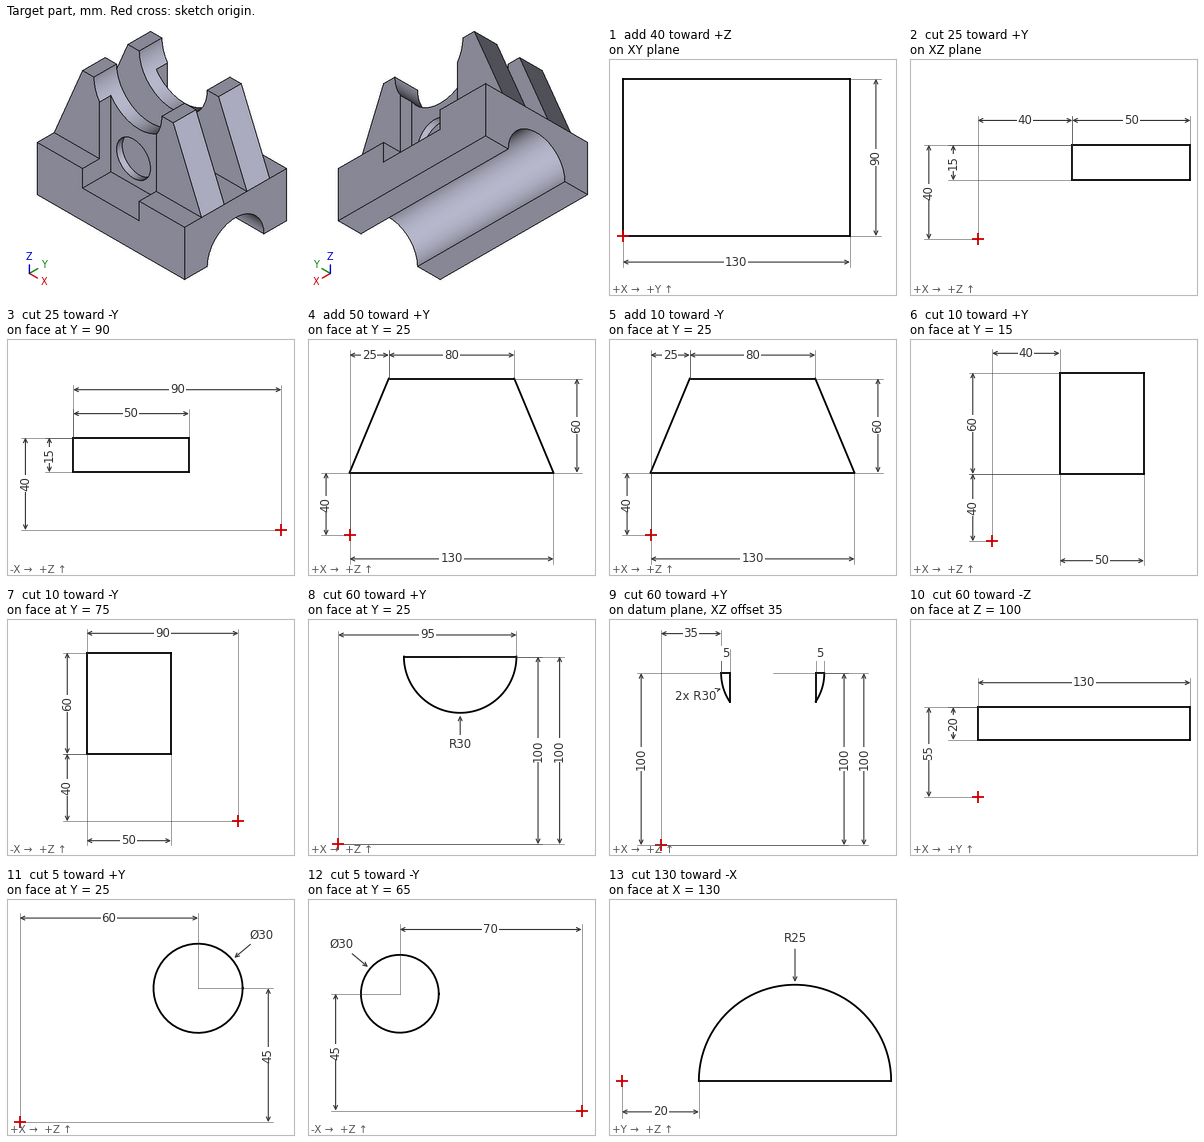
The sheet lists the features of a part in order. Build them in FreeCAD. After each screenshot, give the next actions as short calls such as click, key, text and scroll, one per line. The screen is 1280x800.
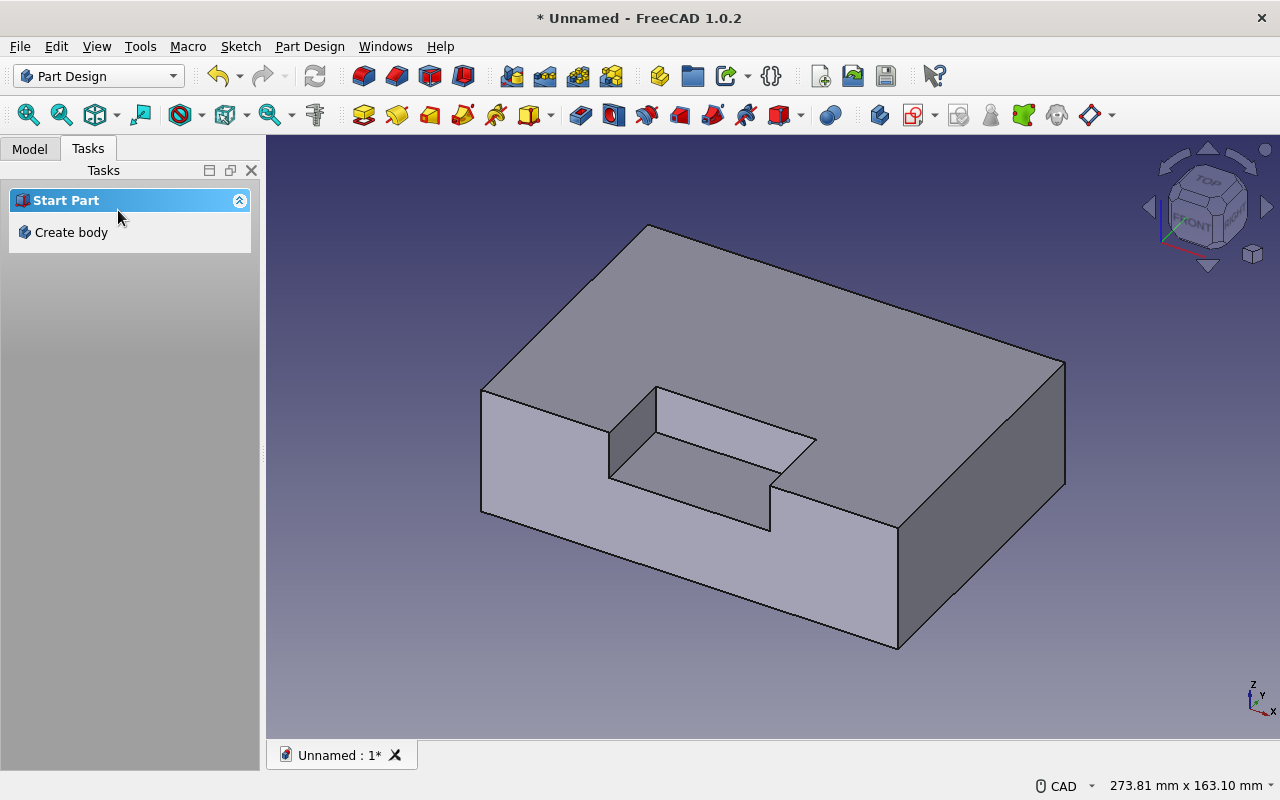
key(4)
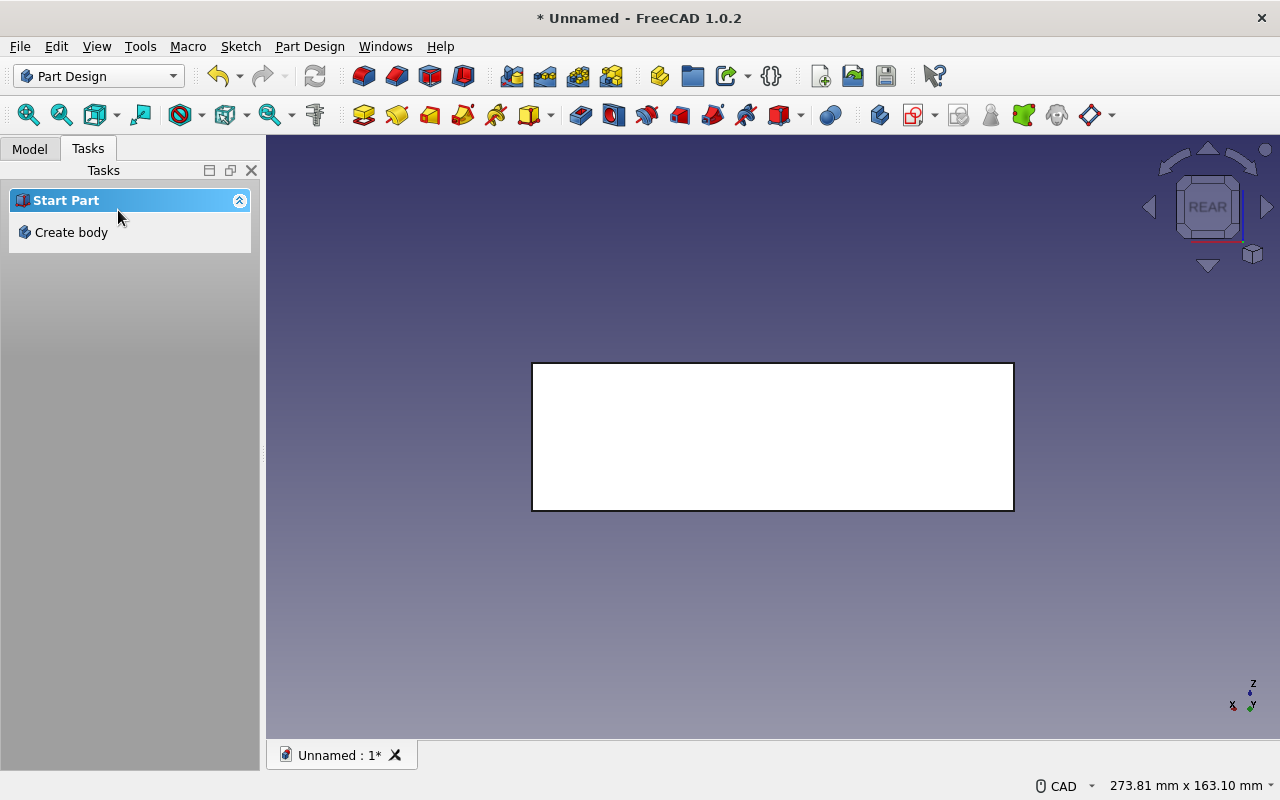
click(635, 436)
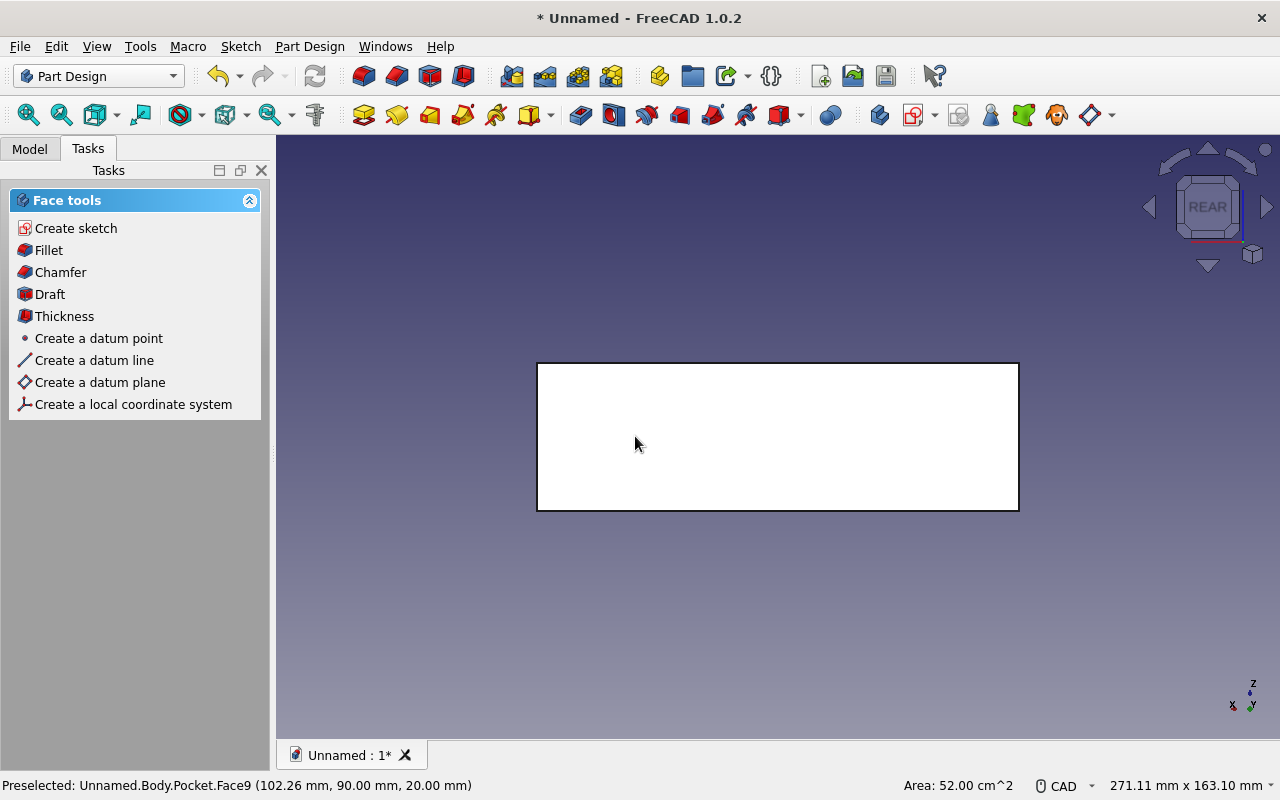
click(912, 116)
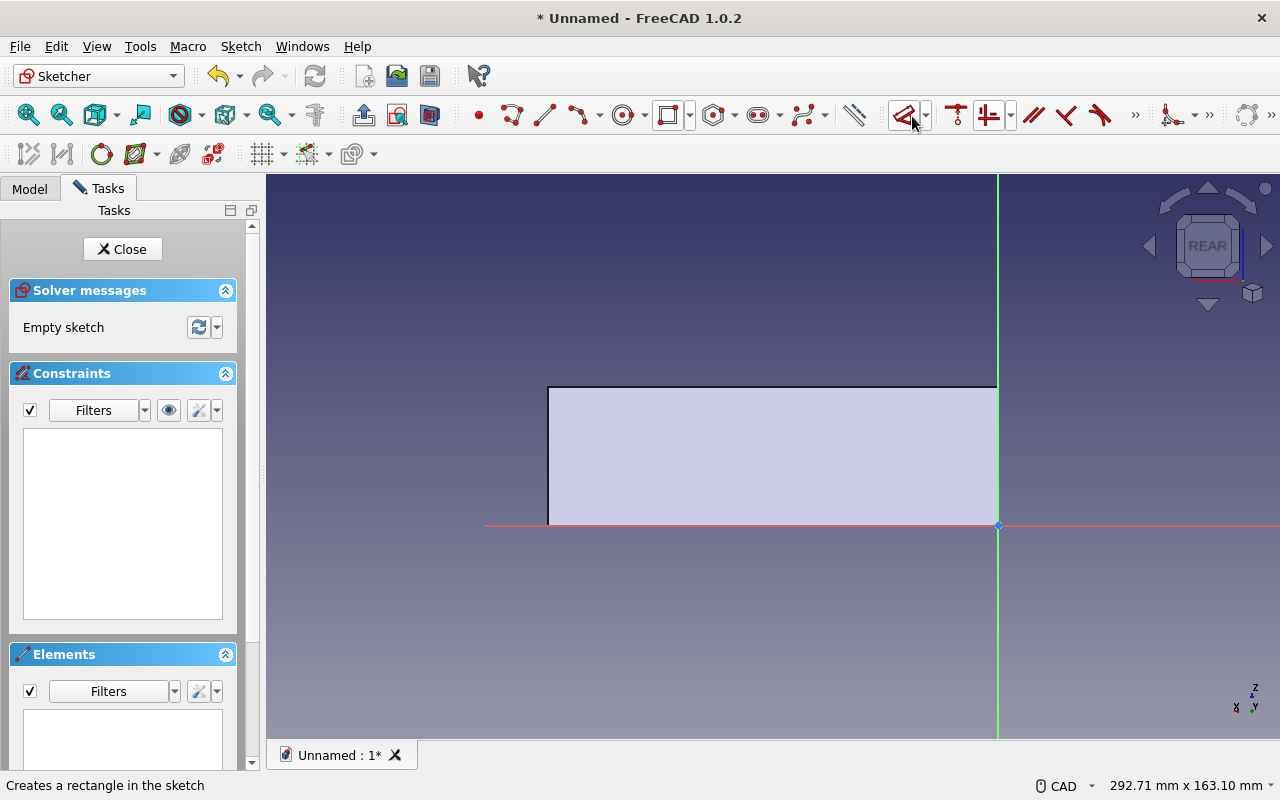
scroll(1010, 456, up, 3)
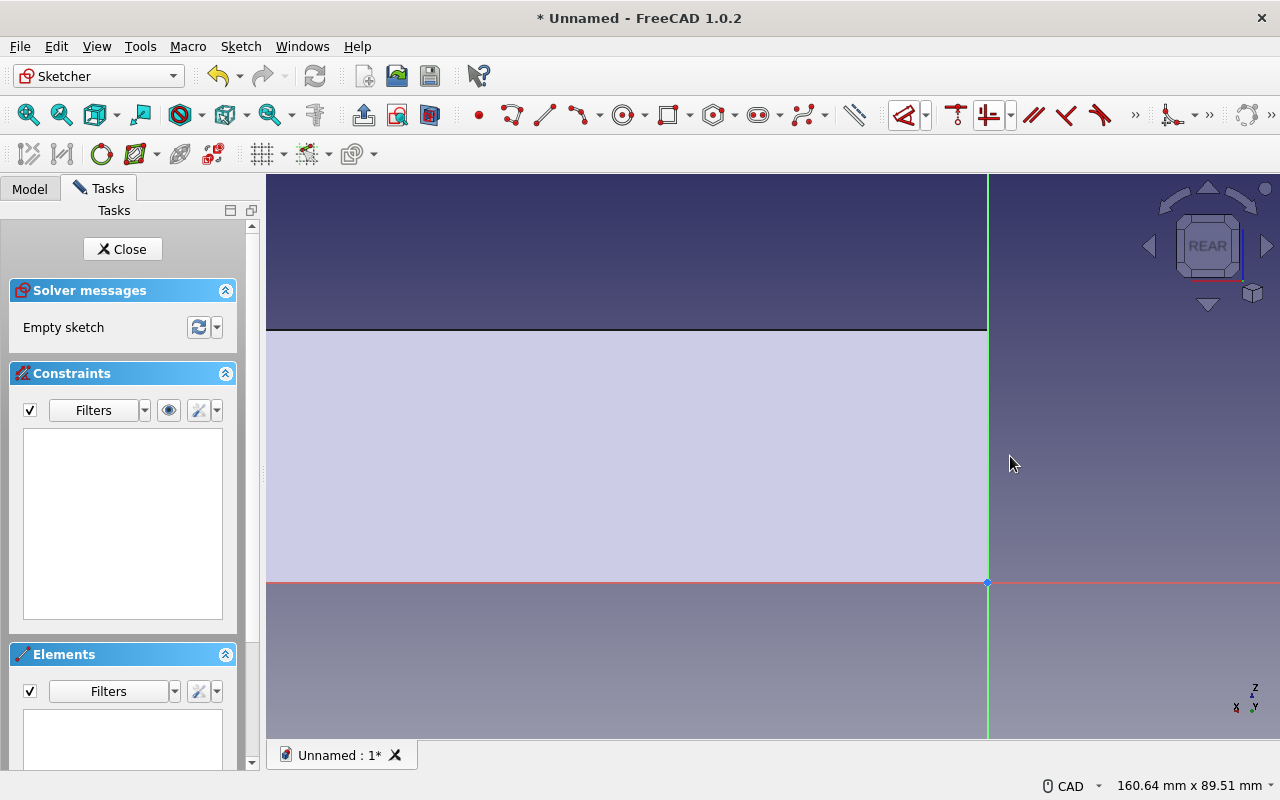
click(668, 116)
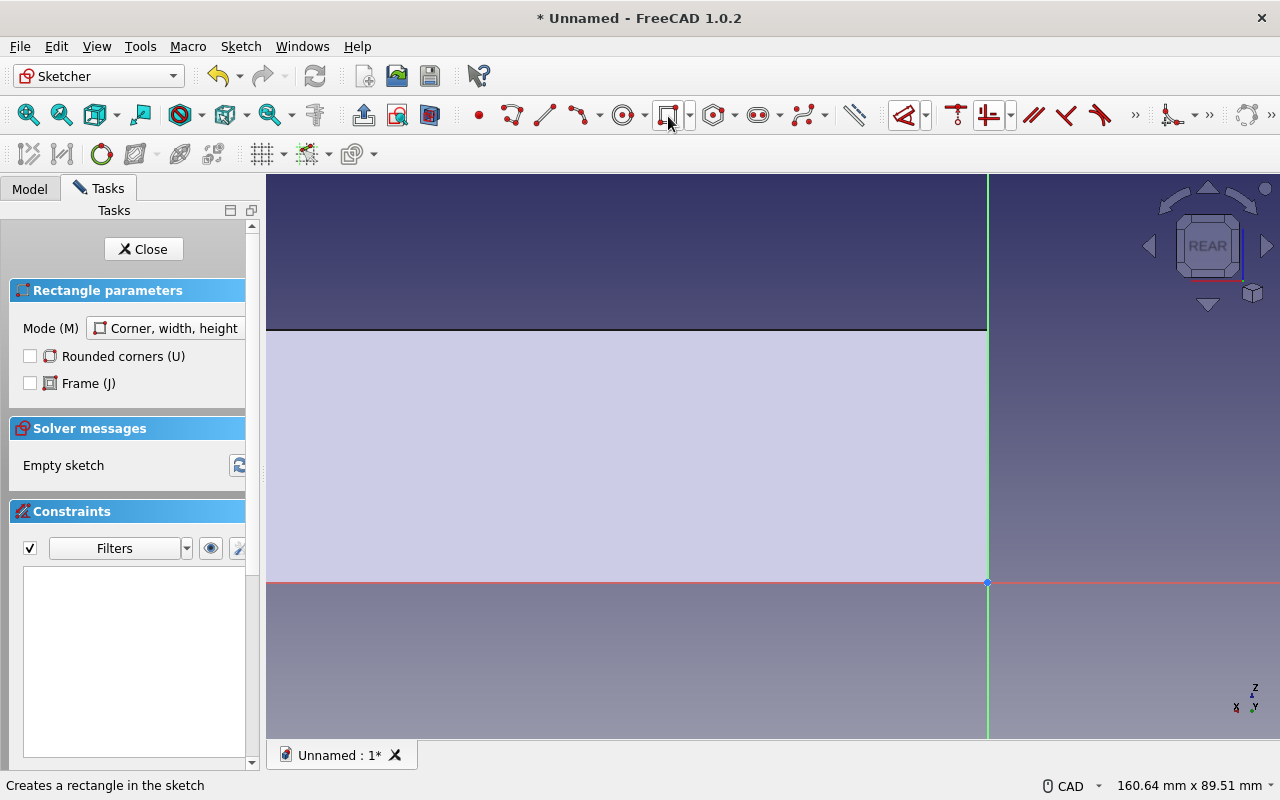
click(420, 330)
click(735, 425)
key(Escape)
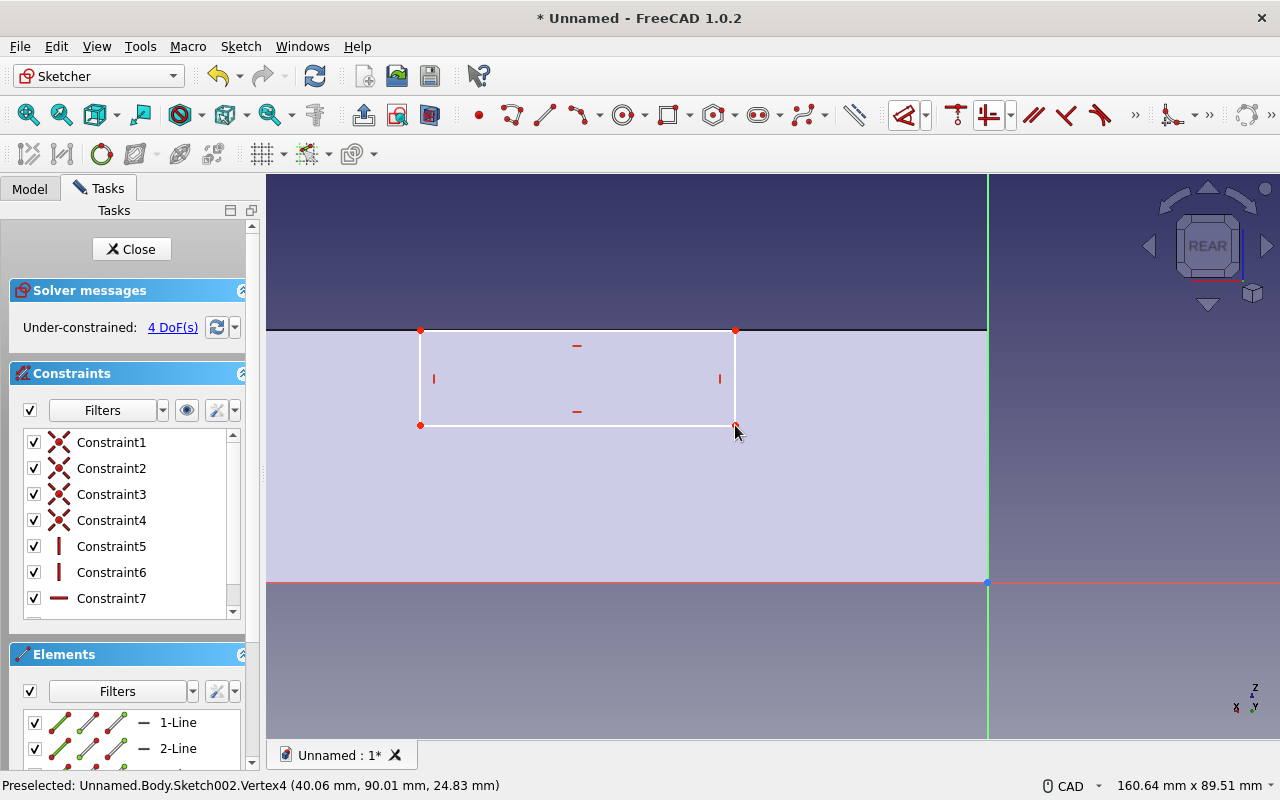
key(d)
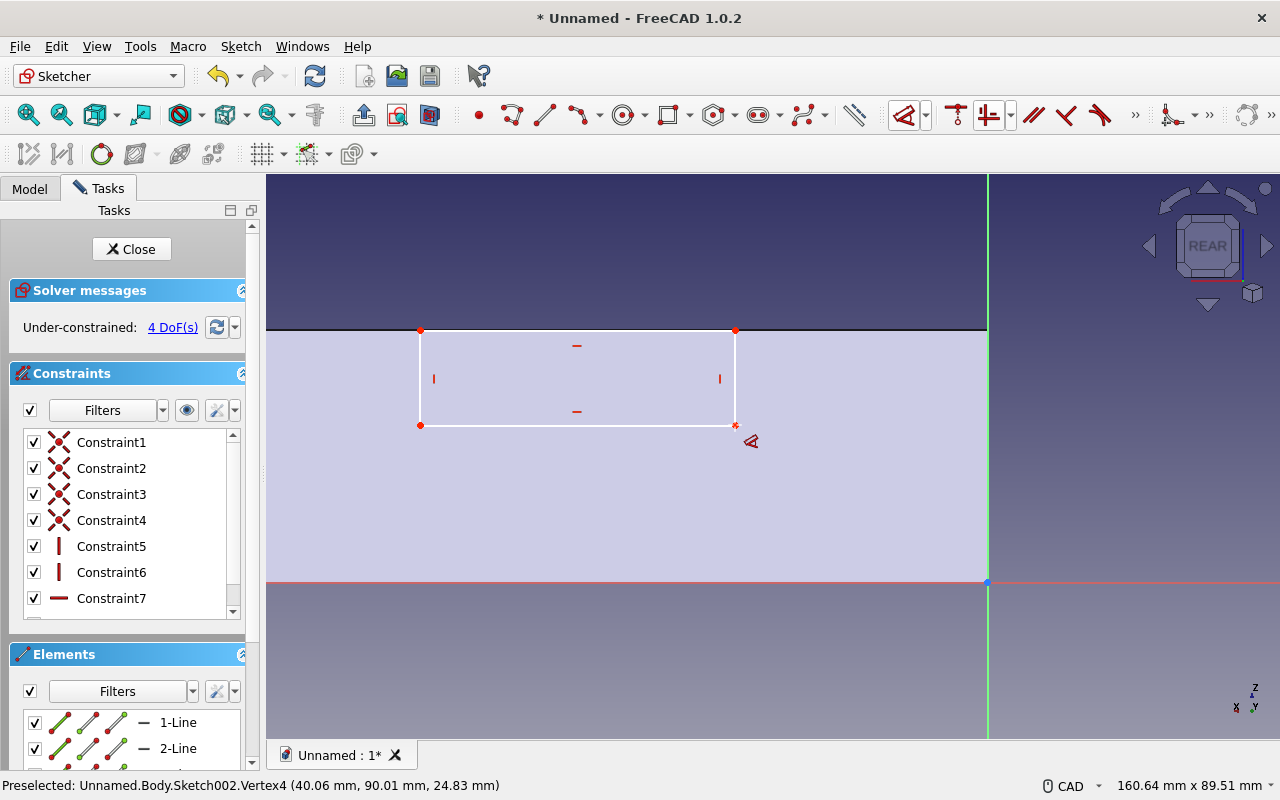
click(420, 359)
click(386, 378)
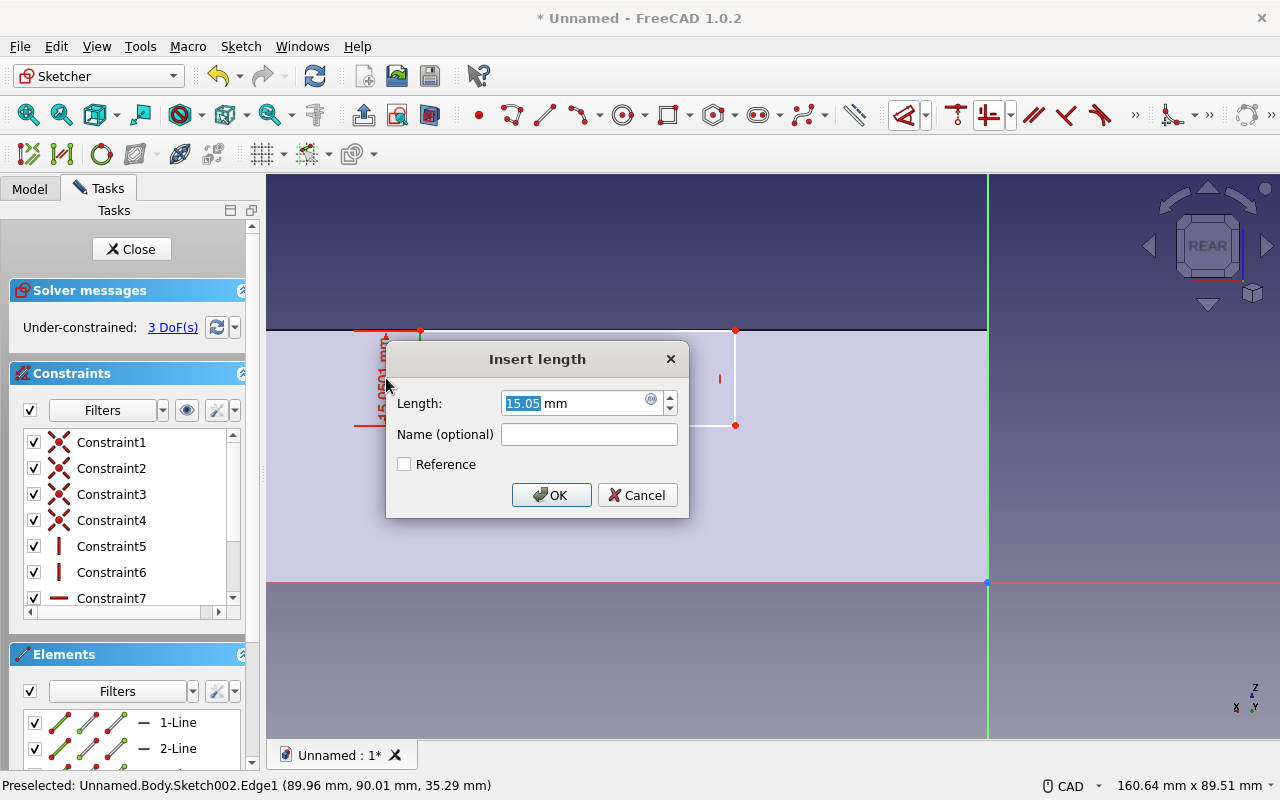
text(15)
key(Return)